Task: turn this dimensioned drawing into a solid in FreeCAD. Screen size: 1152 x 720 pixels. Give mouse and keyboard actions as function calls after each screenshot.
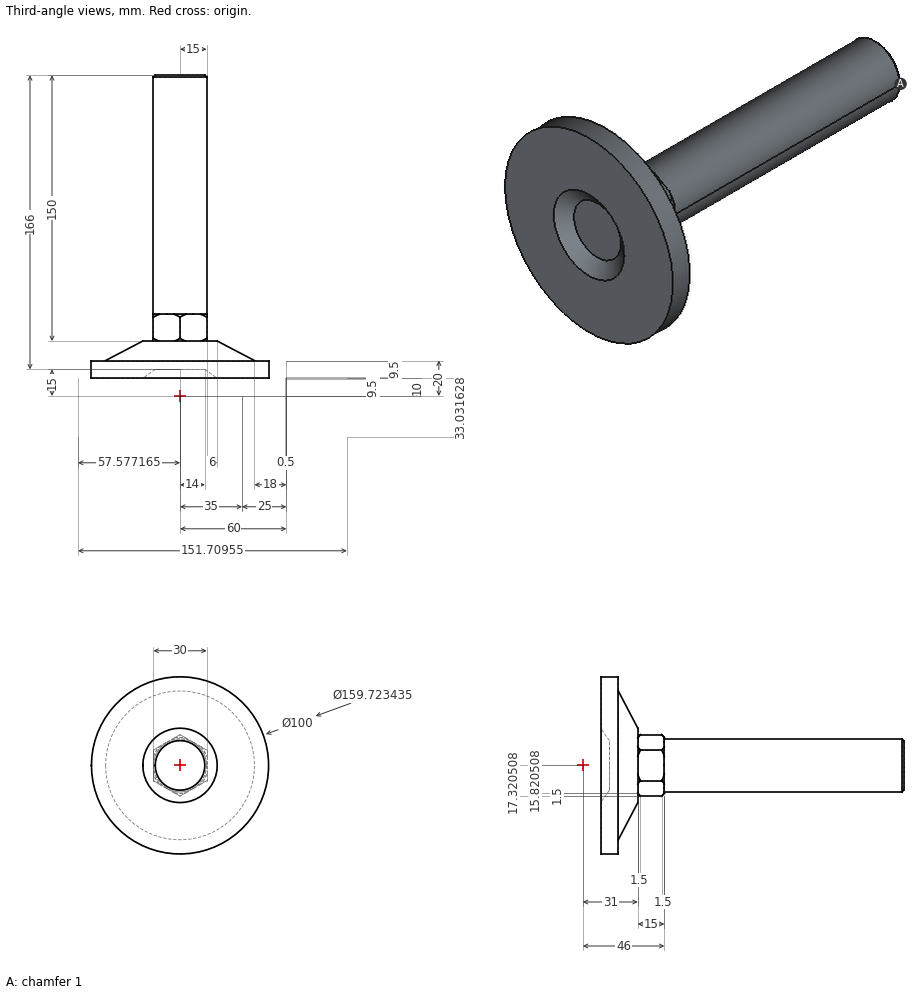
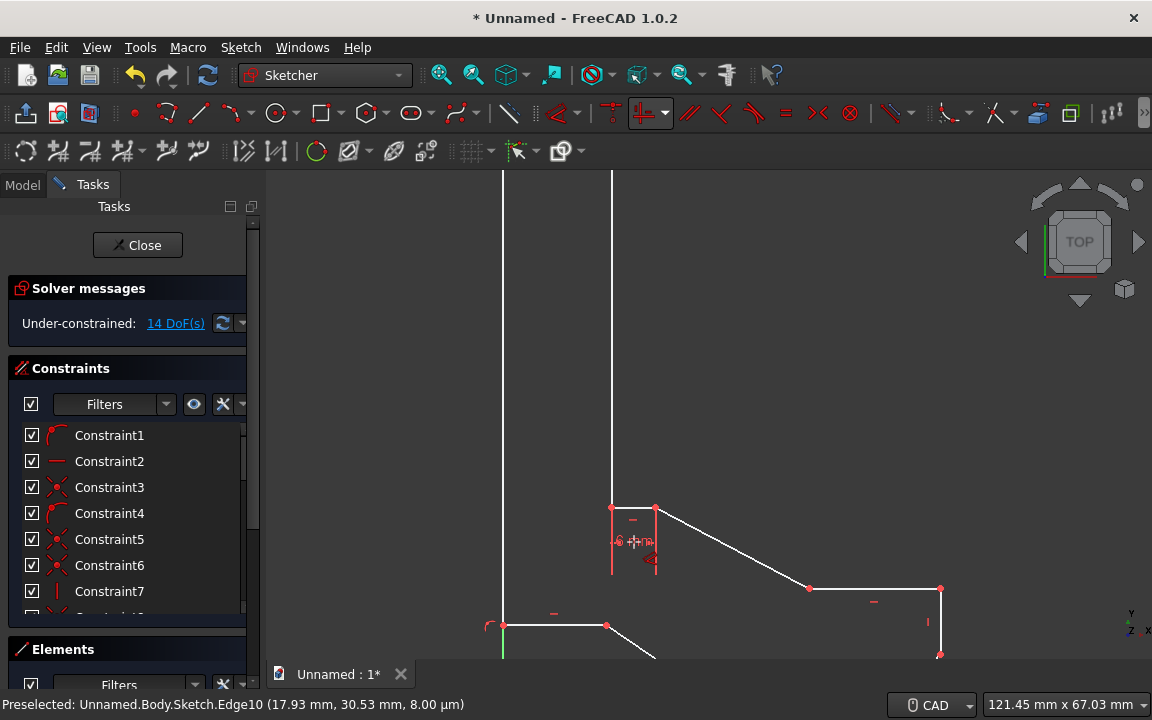
click(534, 625)
click(555, 591)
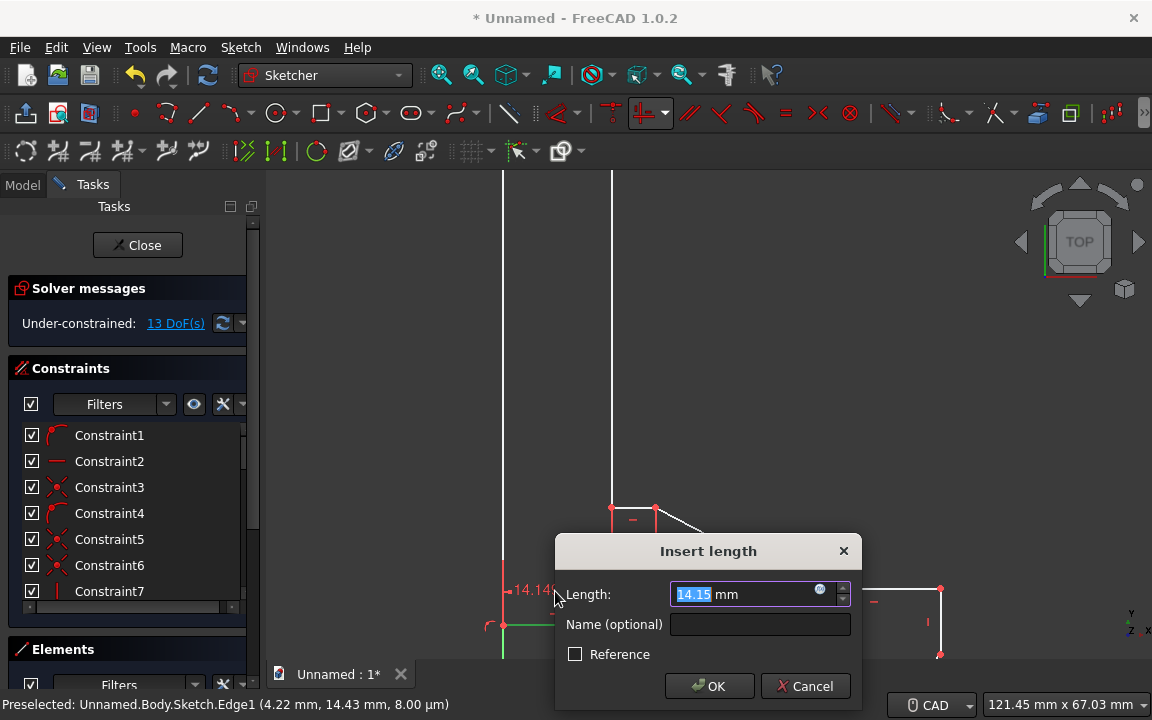
text(14)
key(Return)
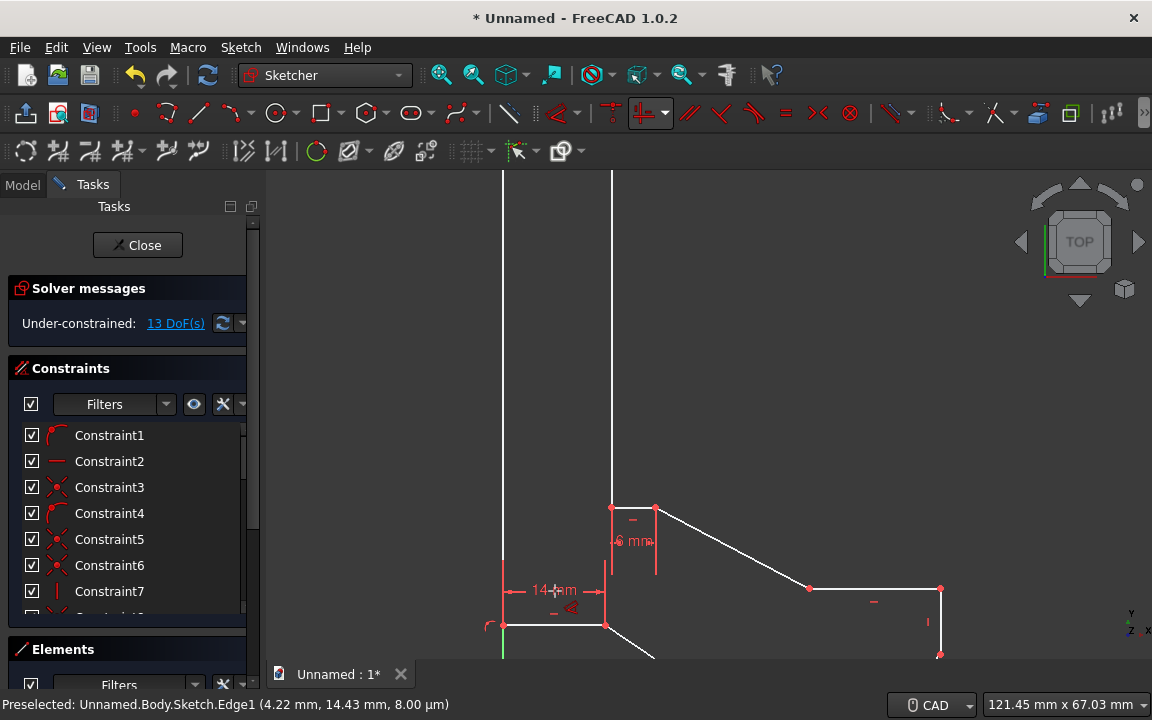
scroll(614, 527, down, 7)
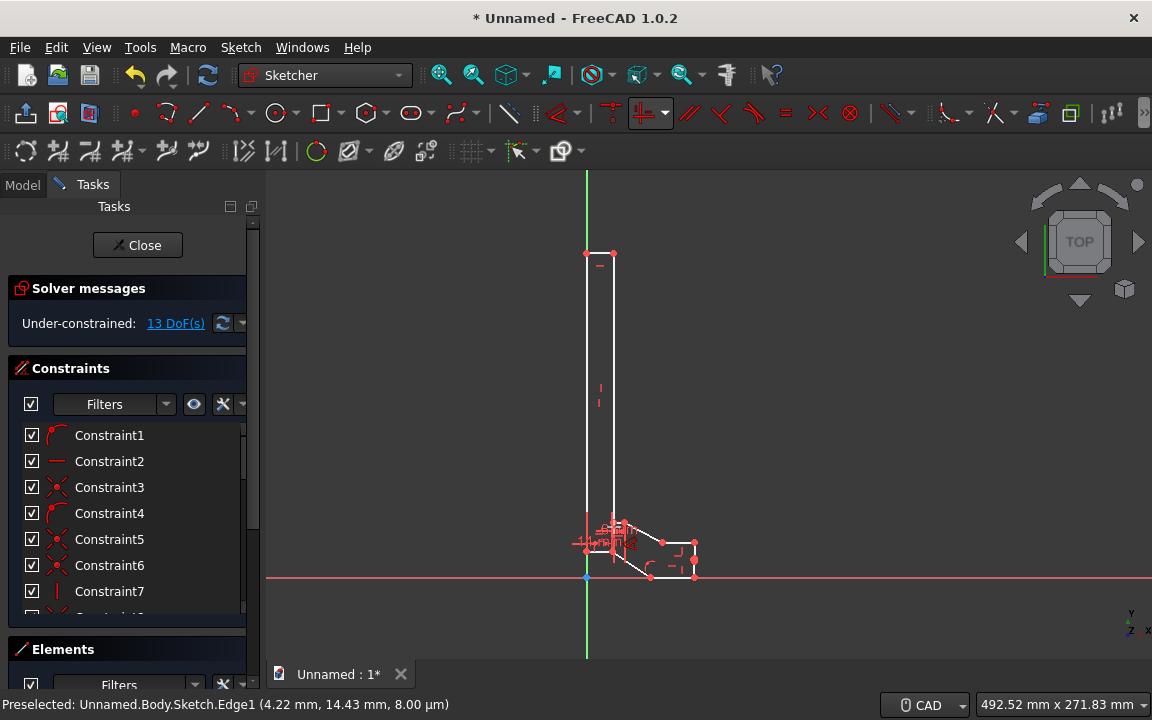
click(664, 578)
click(672, 612)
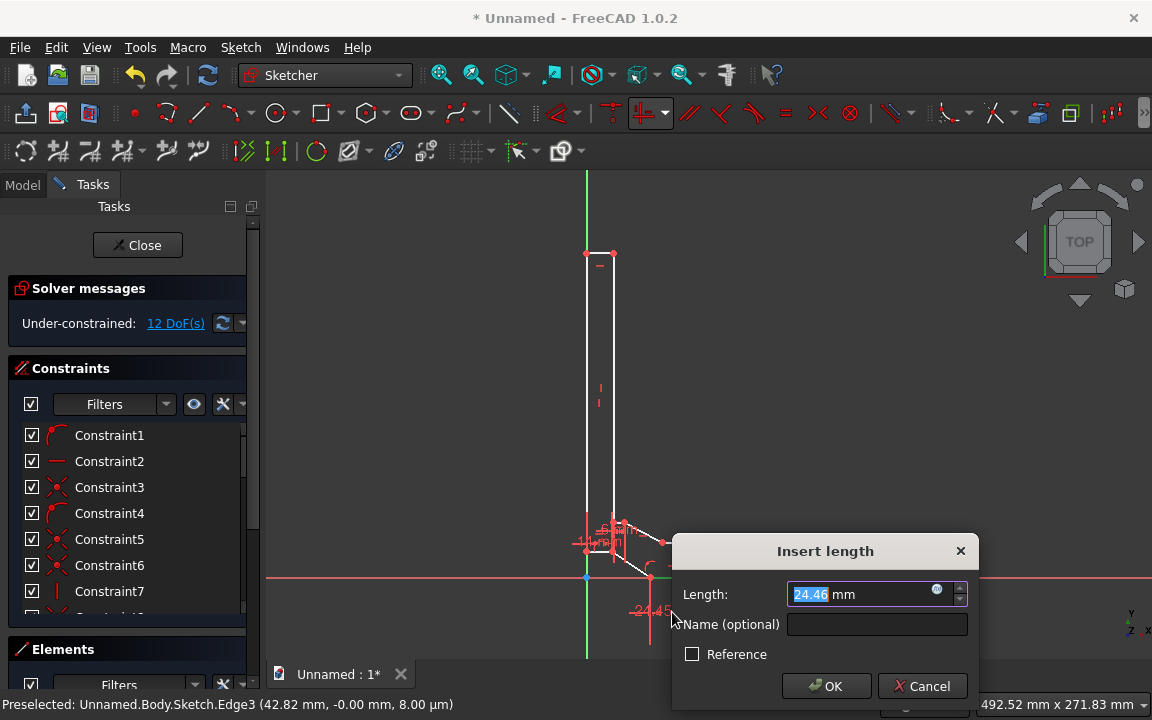
text(25)
key(Return)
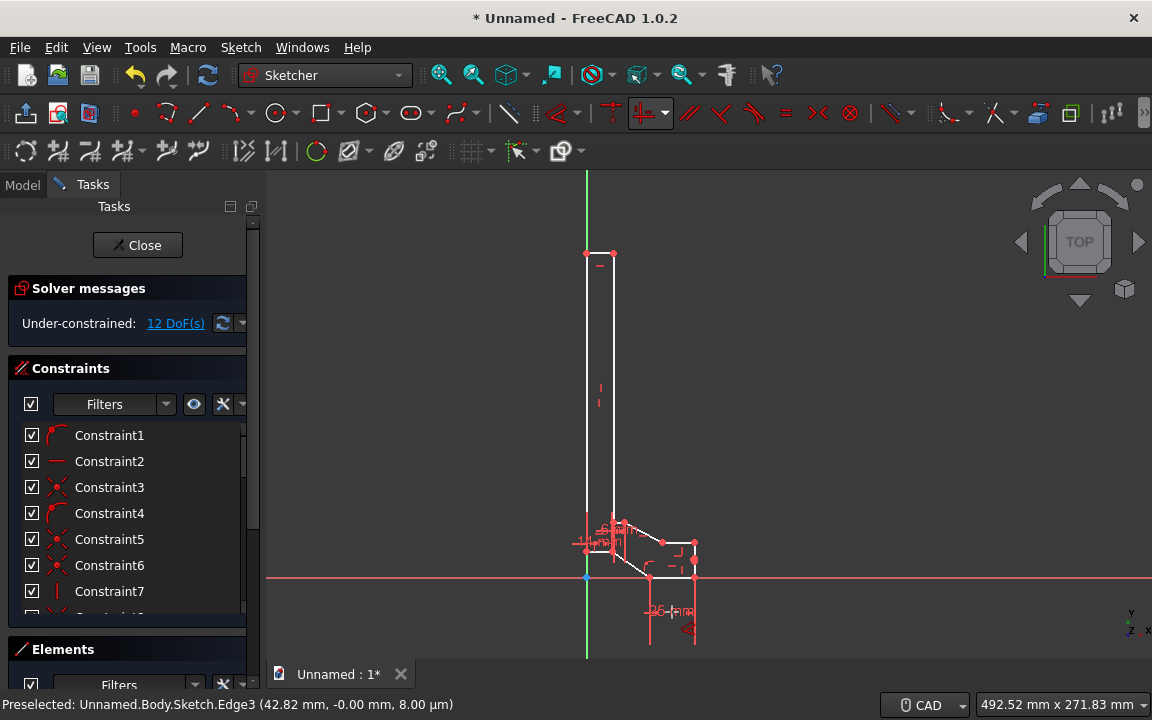
scroll(685, 543, up, 2)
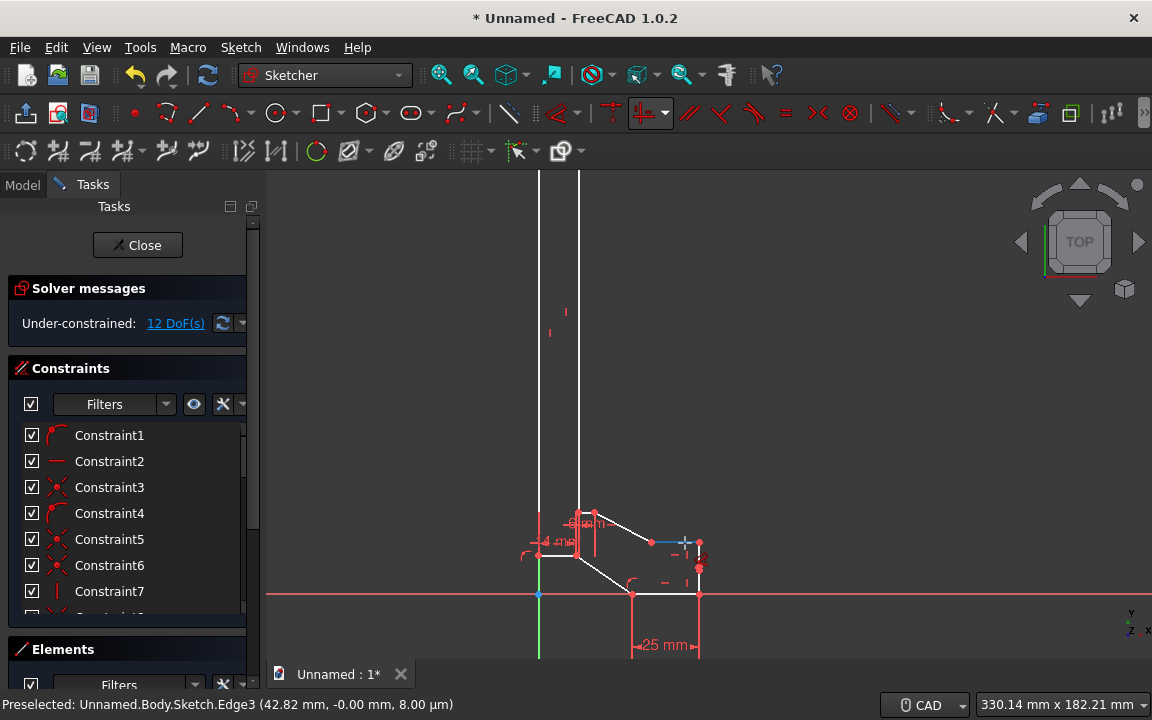
click(685, 542)
click(675, 576)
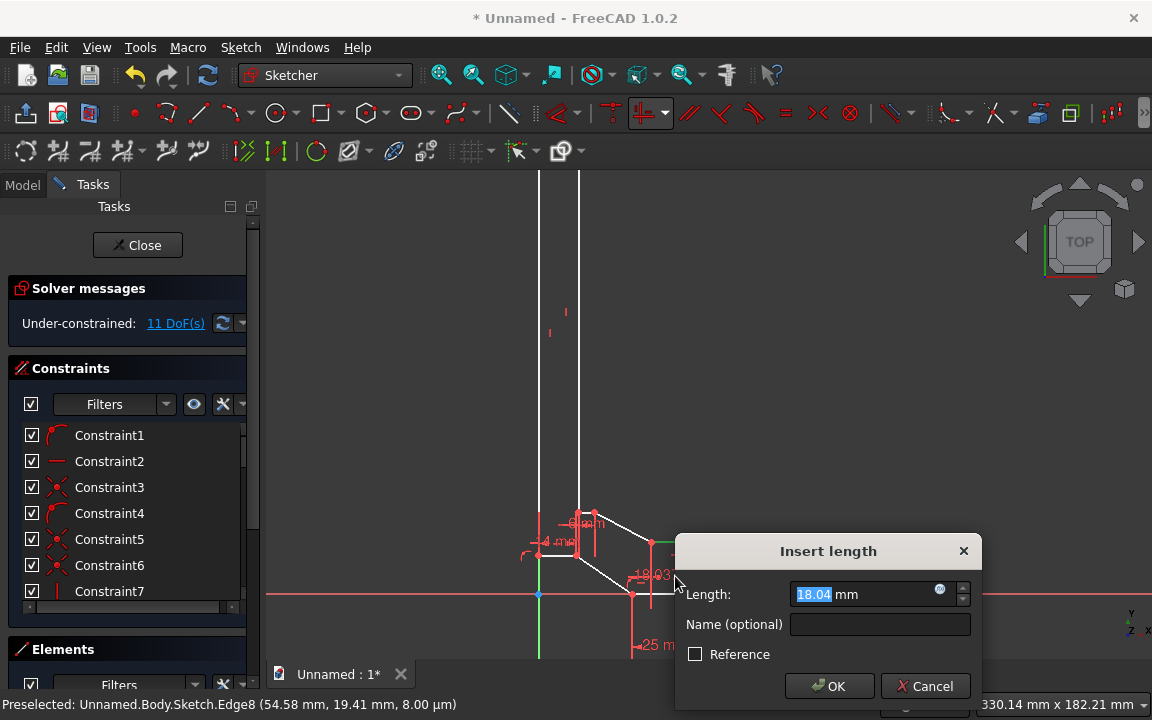
text(18)
key(Return)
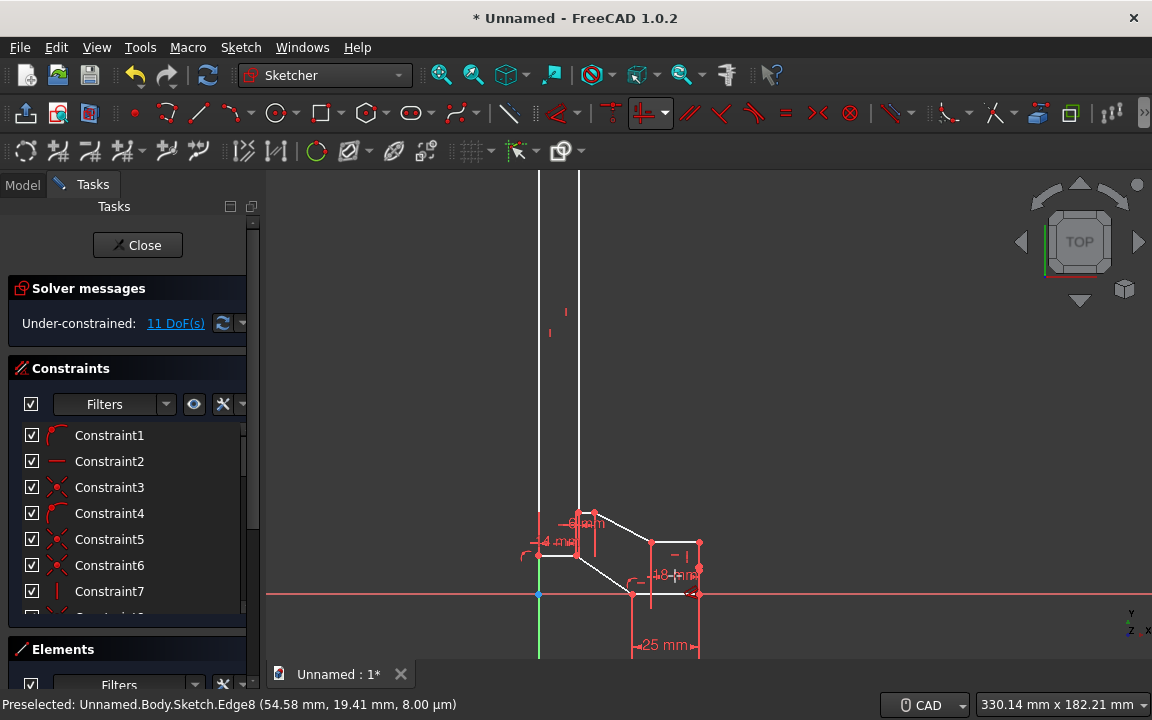
scroll(684, 542, down, 2)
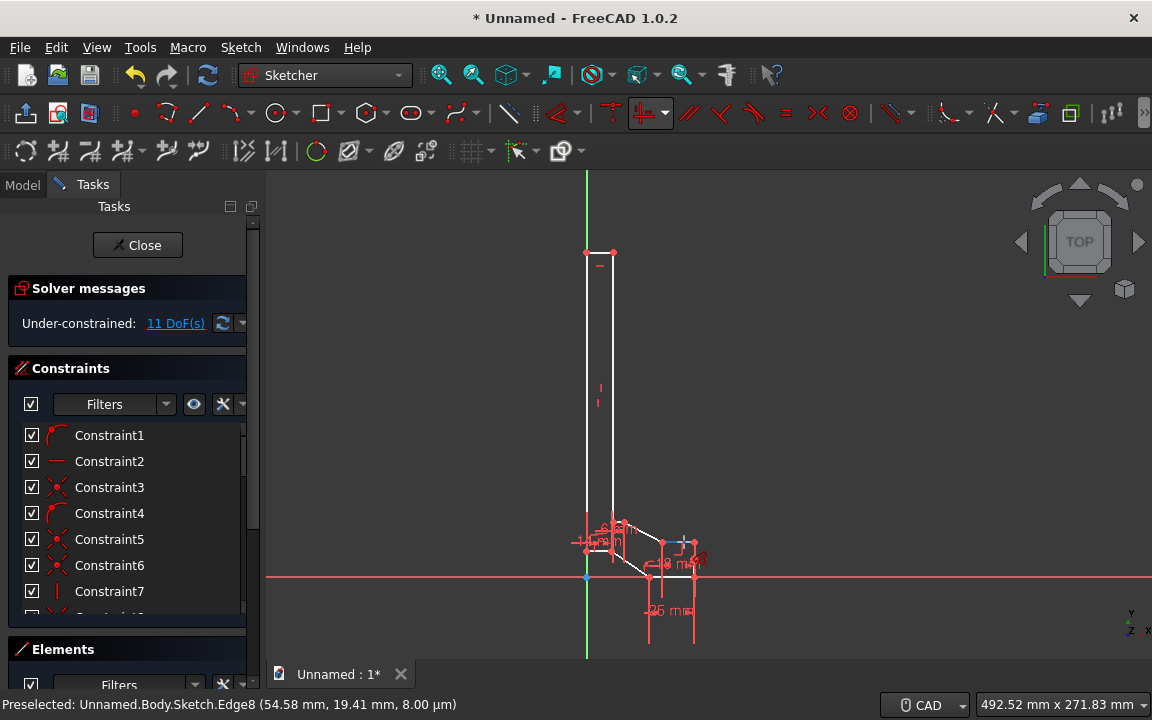
scroll(605, 253, up, 3)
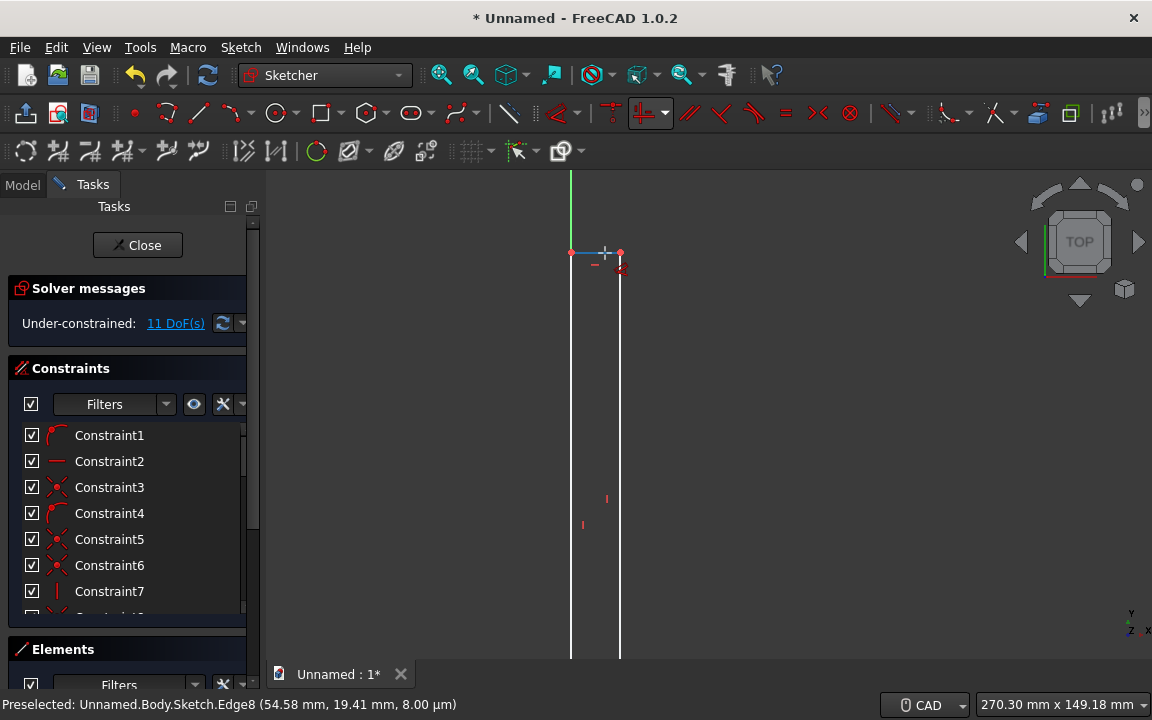
click(605, 253)
click(596, 219)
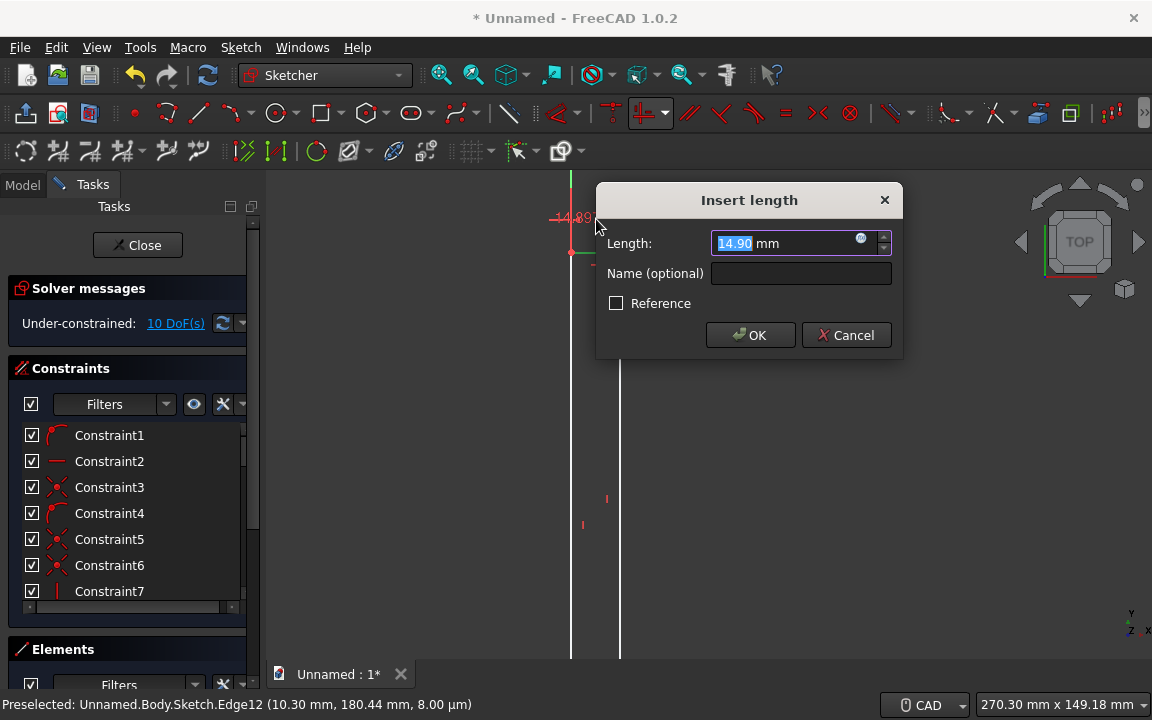
text(15)
key(Return)